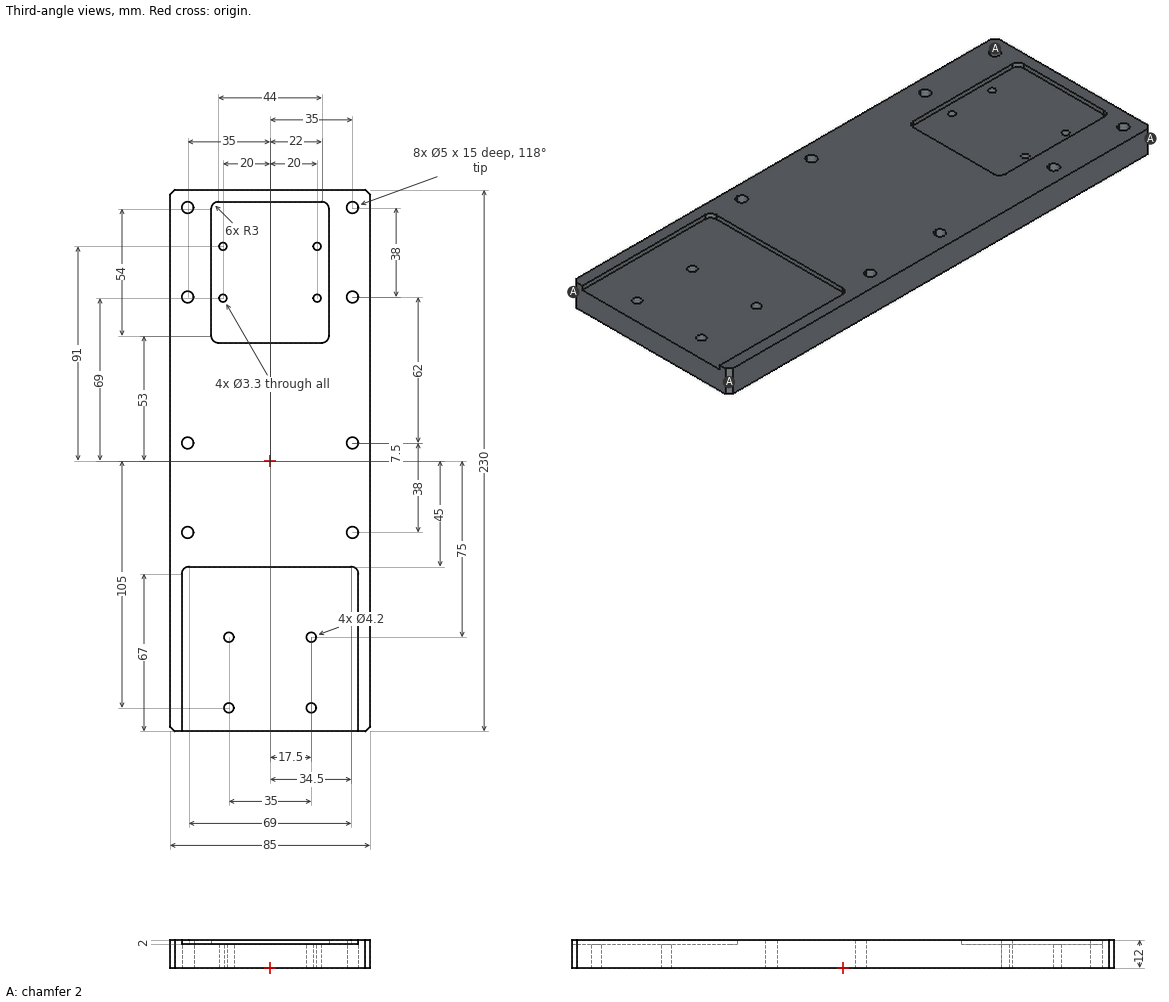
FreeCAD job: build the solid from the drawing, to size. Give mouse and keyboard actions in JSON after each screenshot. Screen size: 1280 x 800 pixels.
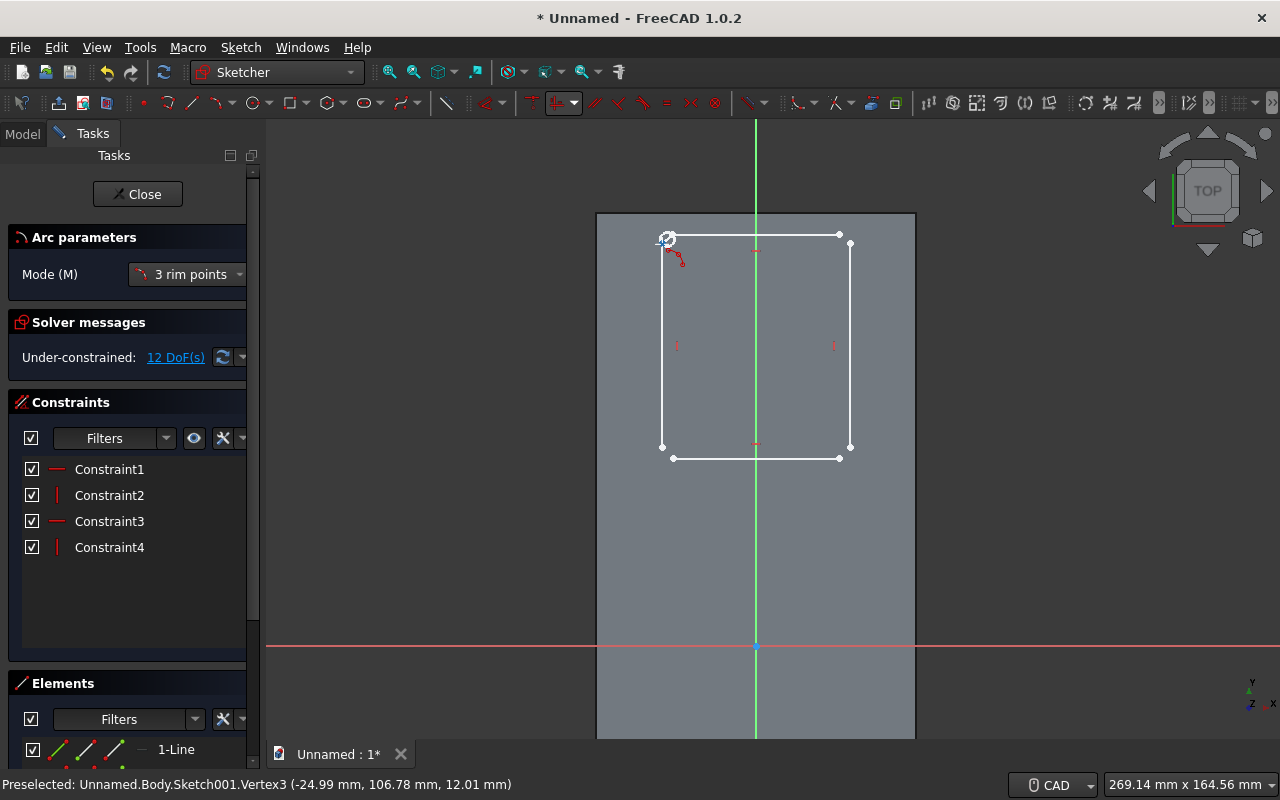
{"action": "scroll", "coordinate": [665, 235], "scroll_direction": "up", "scroll_amount": 8}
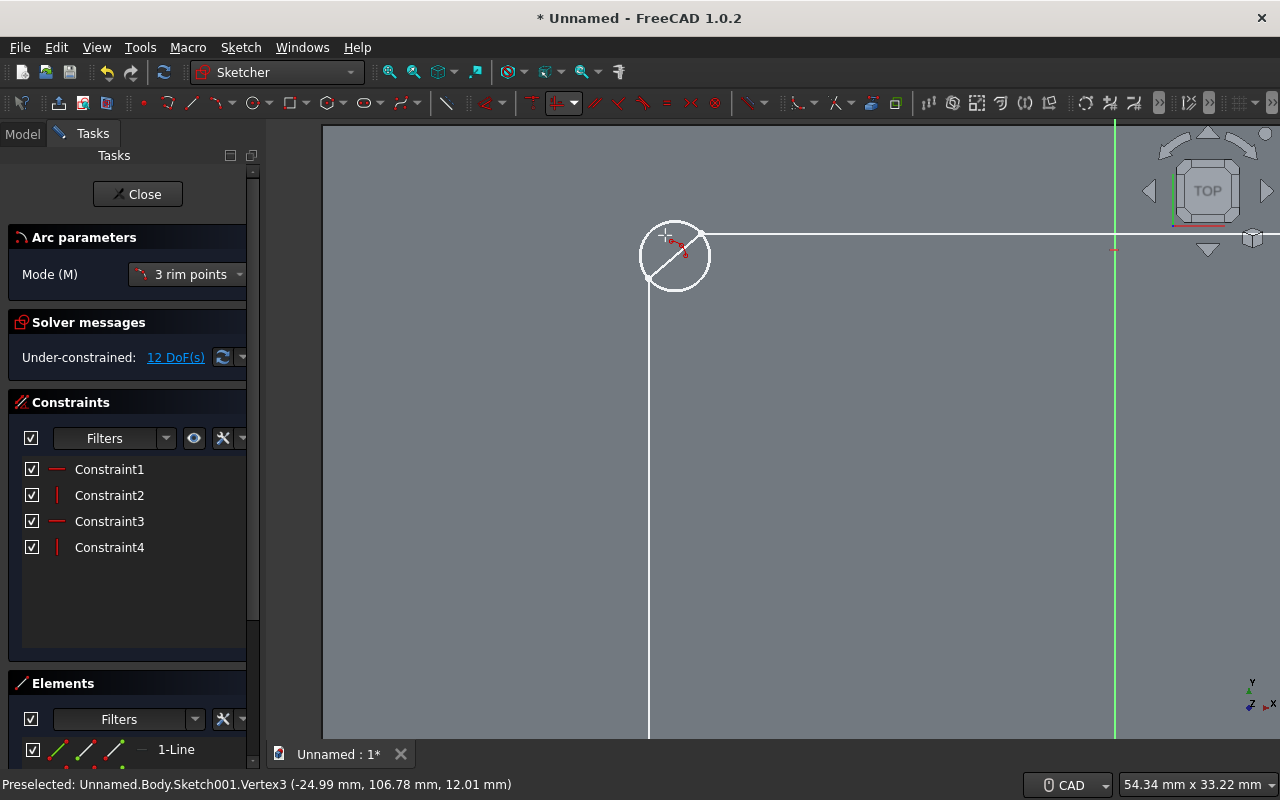
{"action": "left_click", "coordinate": [665, 235]}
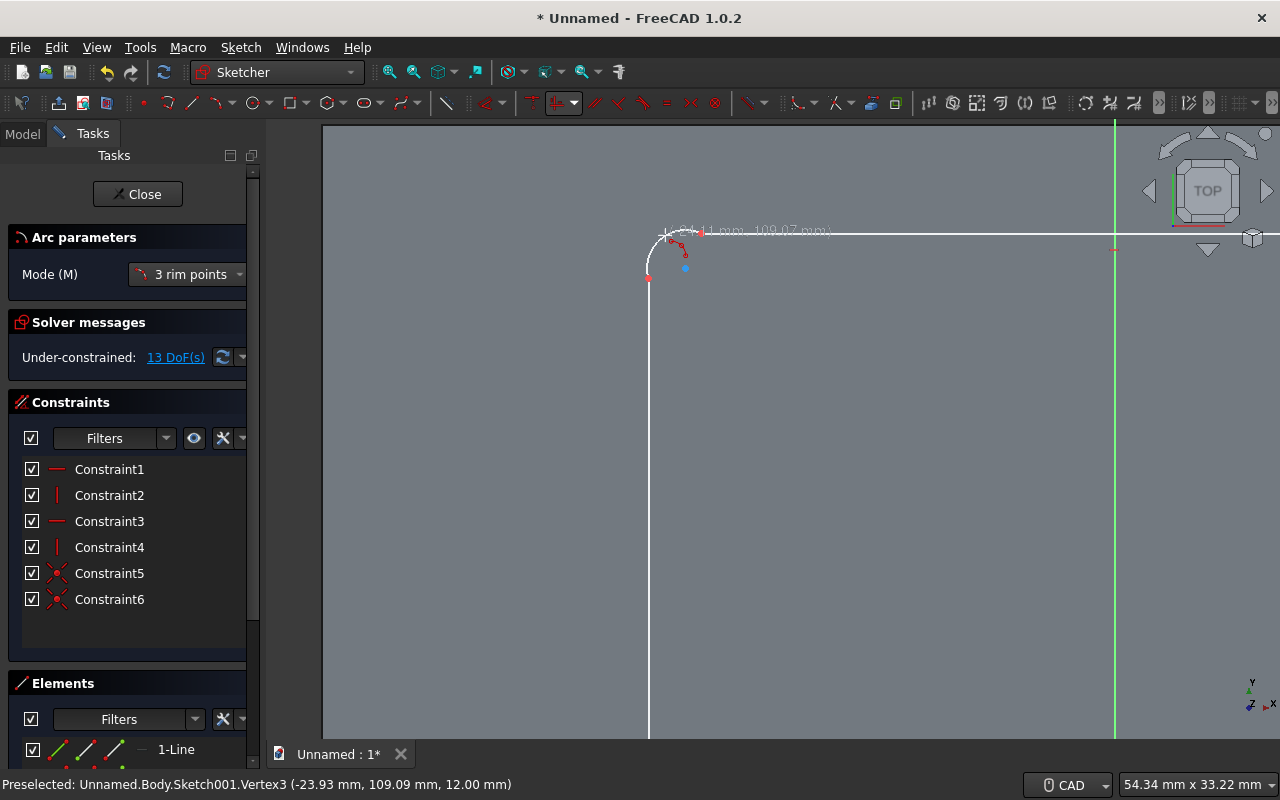
{"action": "scroll", "coordinate": [664, 241], "scroll_direction": "down", "scroll_amount": 12}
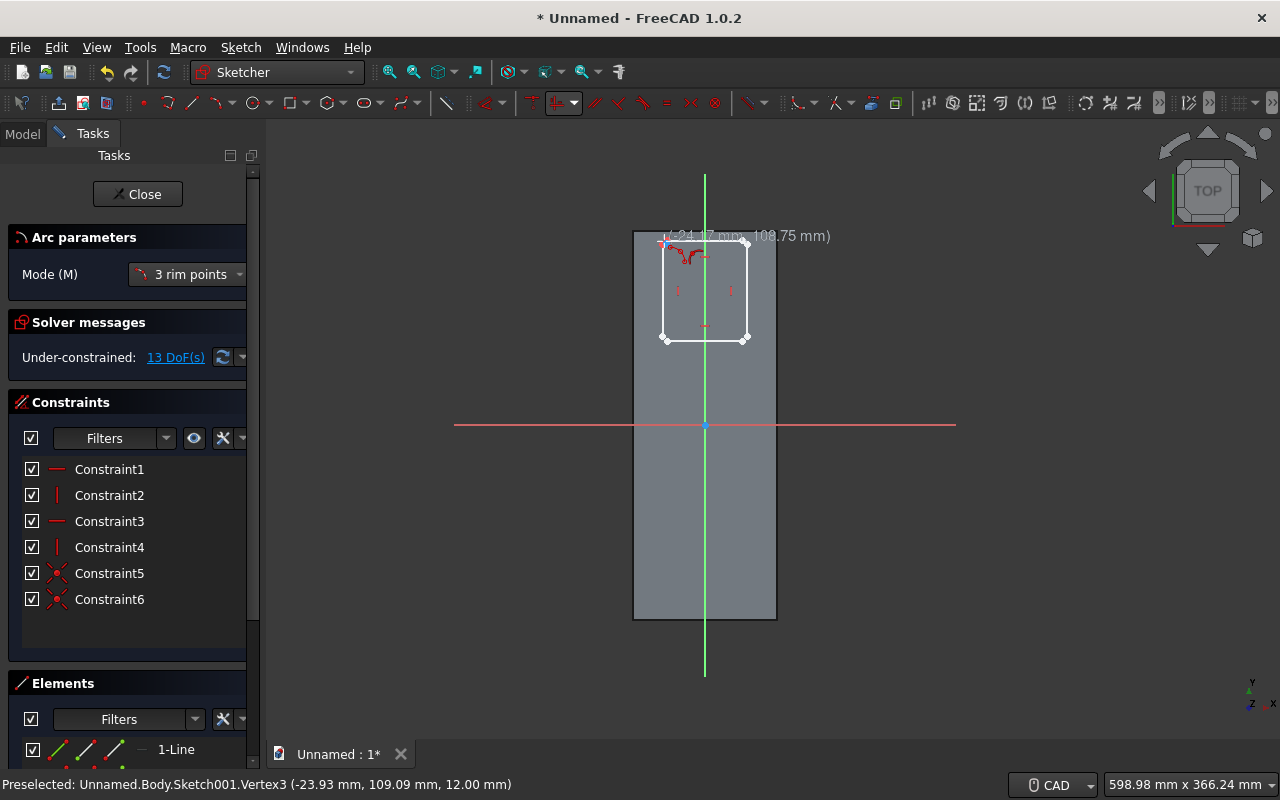
{"action": "scroll", "coordinate": [663, 336], "scroll_direction": "up", "scroll_amount": 4}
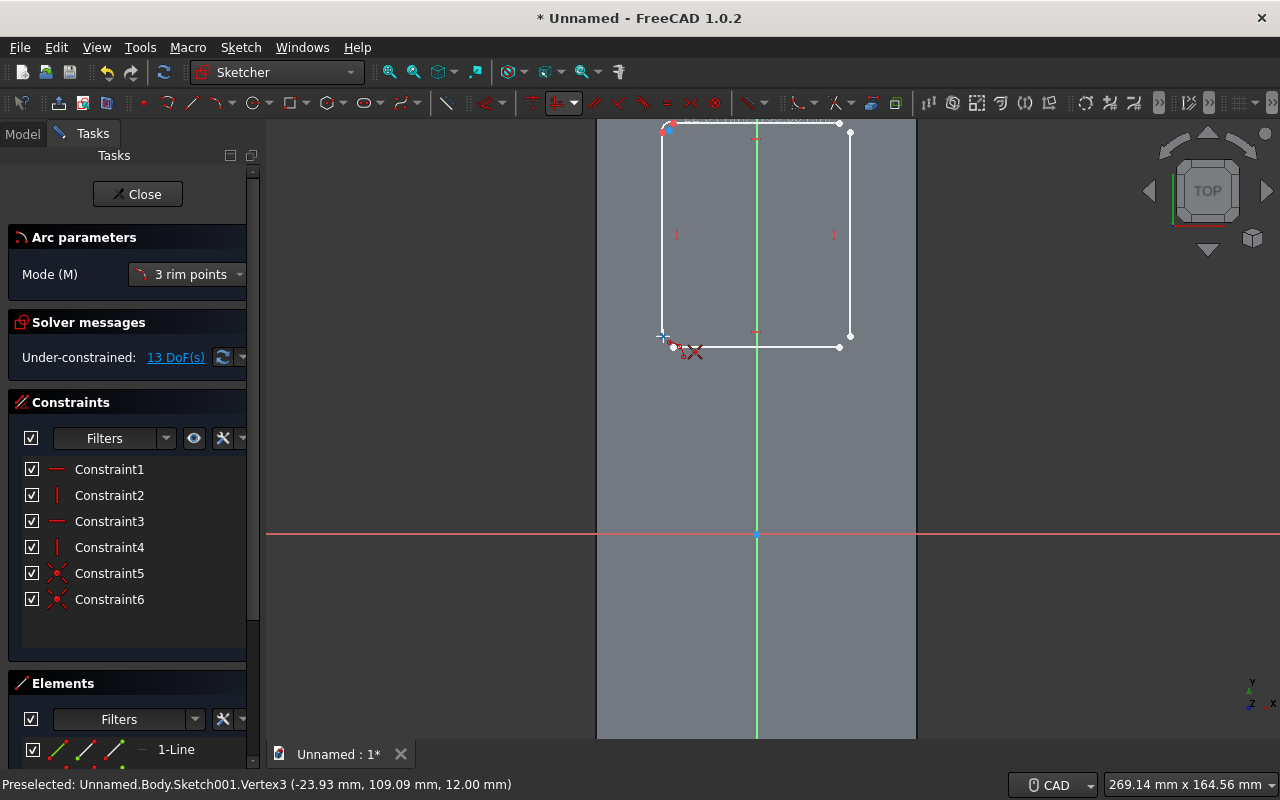
{"action": "left_click", "coordinate": [662, 336]}
{"action": "left_click", "coordinate": [673, 347]}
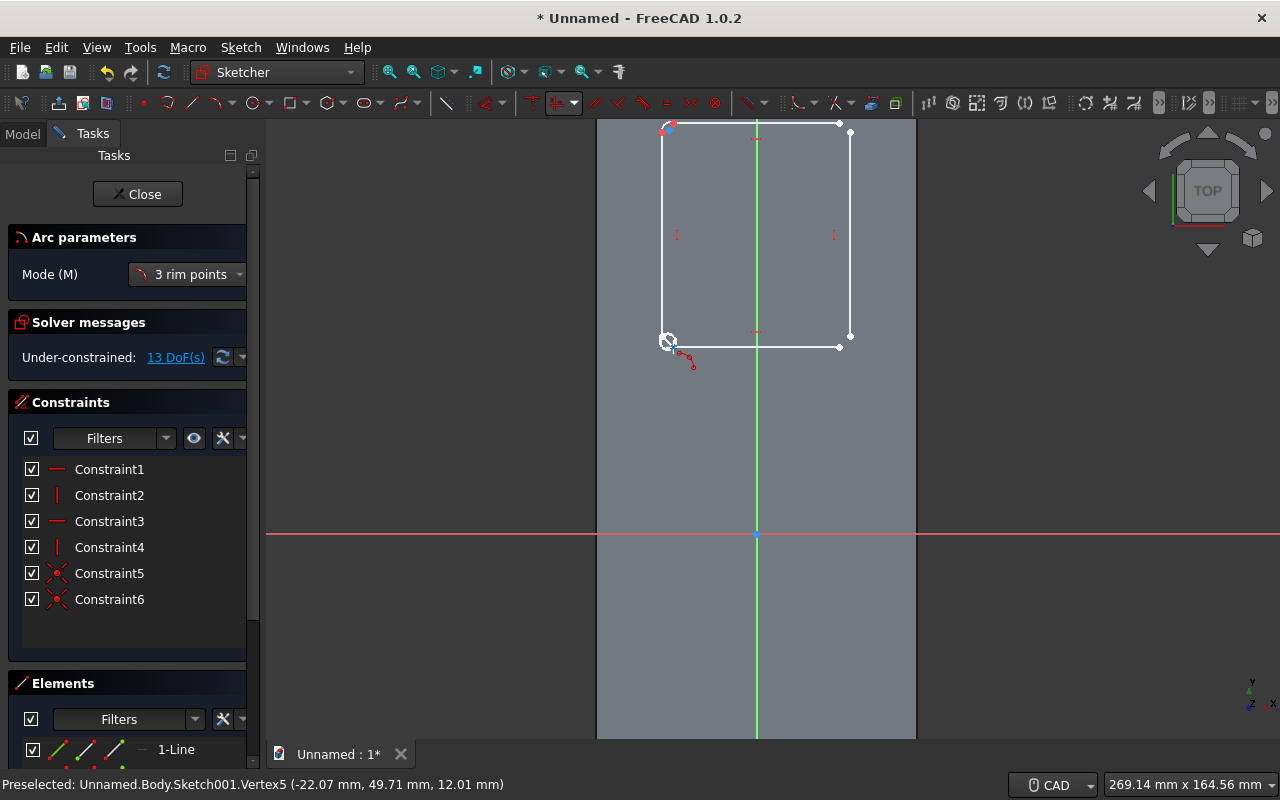
{"action": "scroll", "coordinate": [666, 343], "scroll_direction": "up", "scroll_amount": 8}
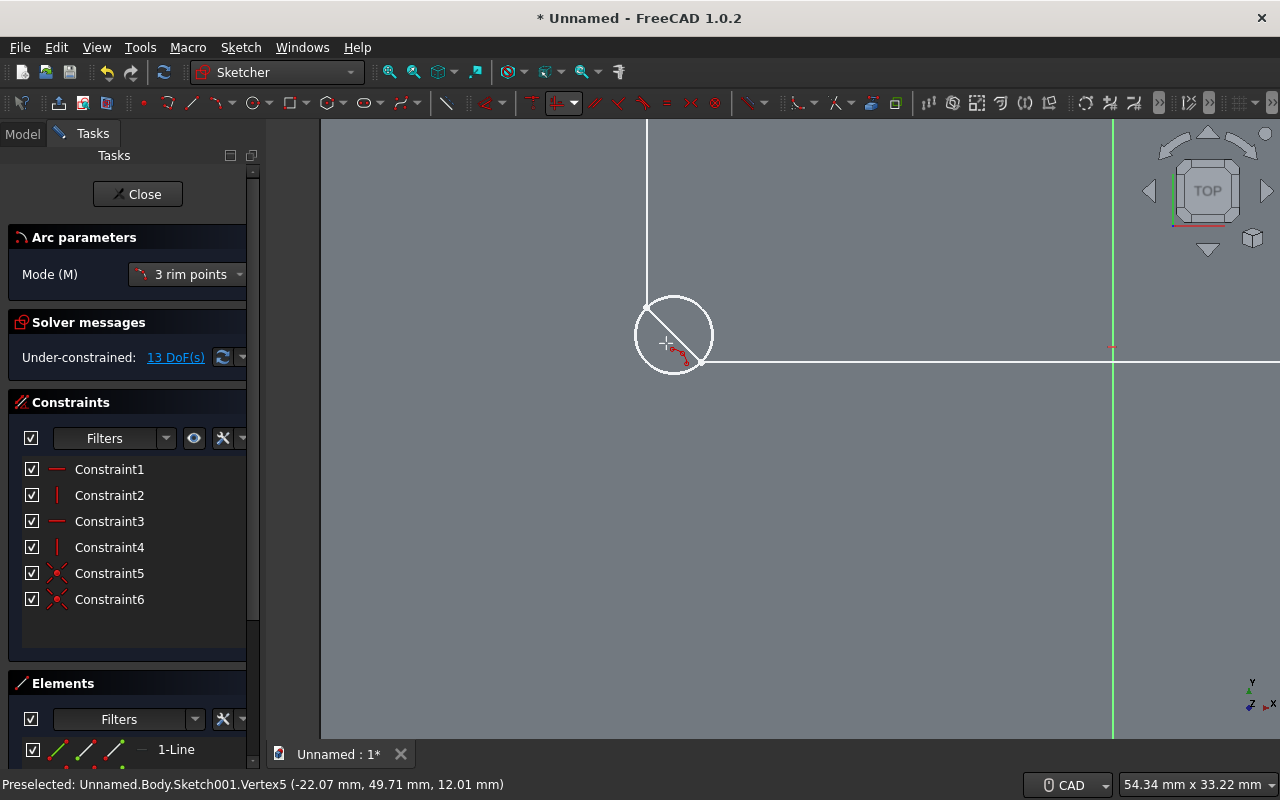
{"action": "left_click", "coordinate": [663, 340]}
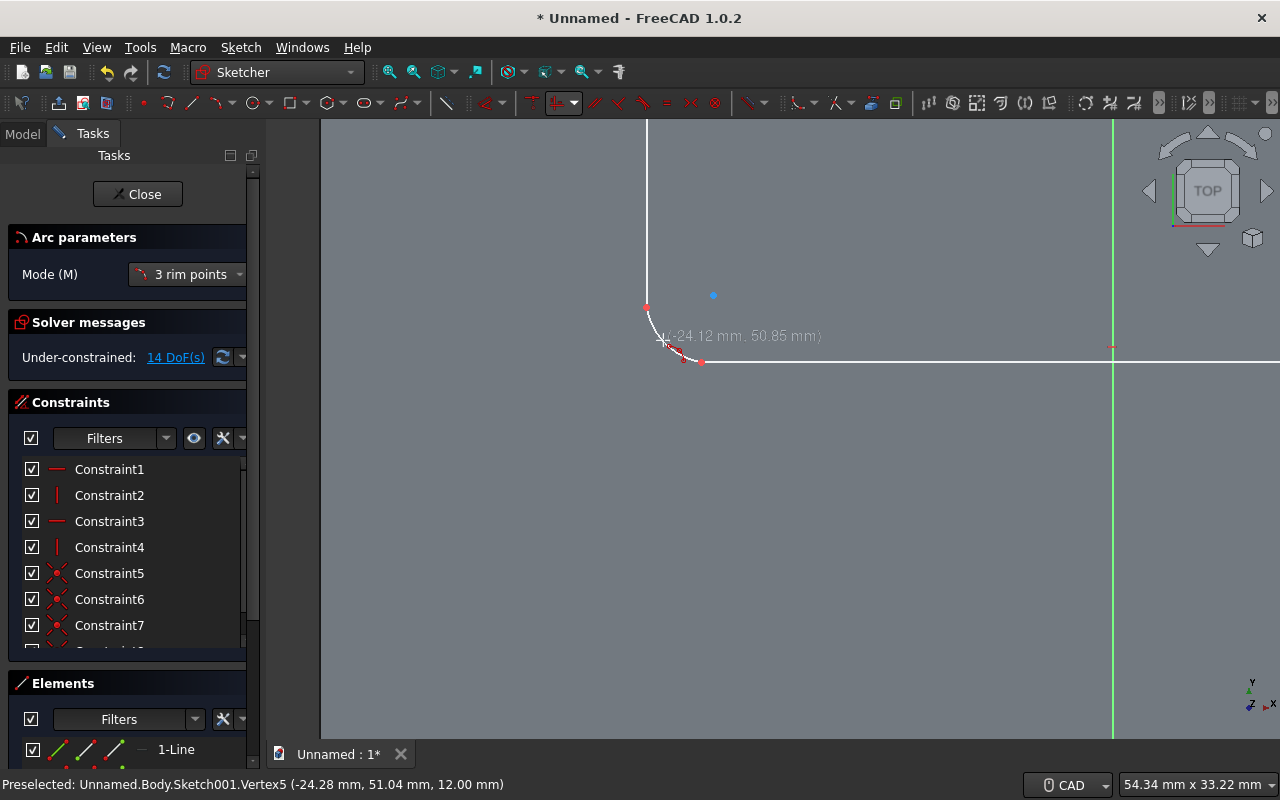
{"action": "scroll", "coordinate": [664, 338], "scroll_direction": "down", "scroll_amount": 12}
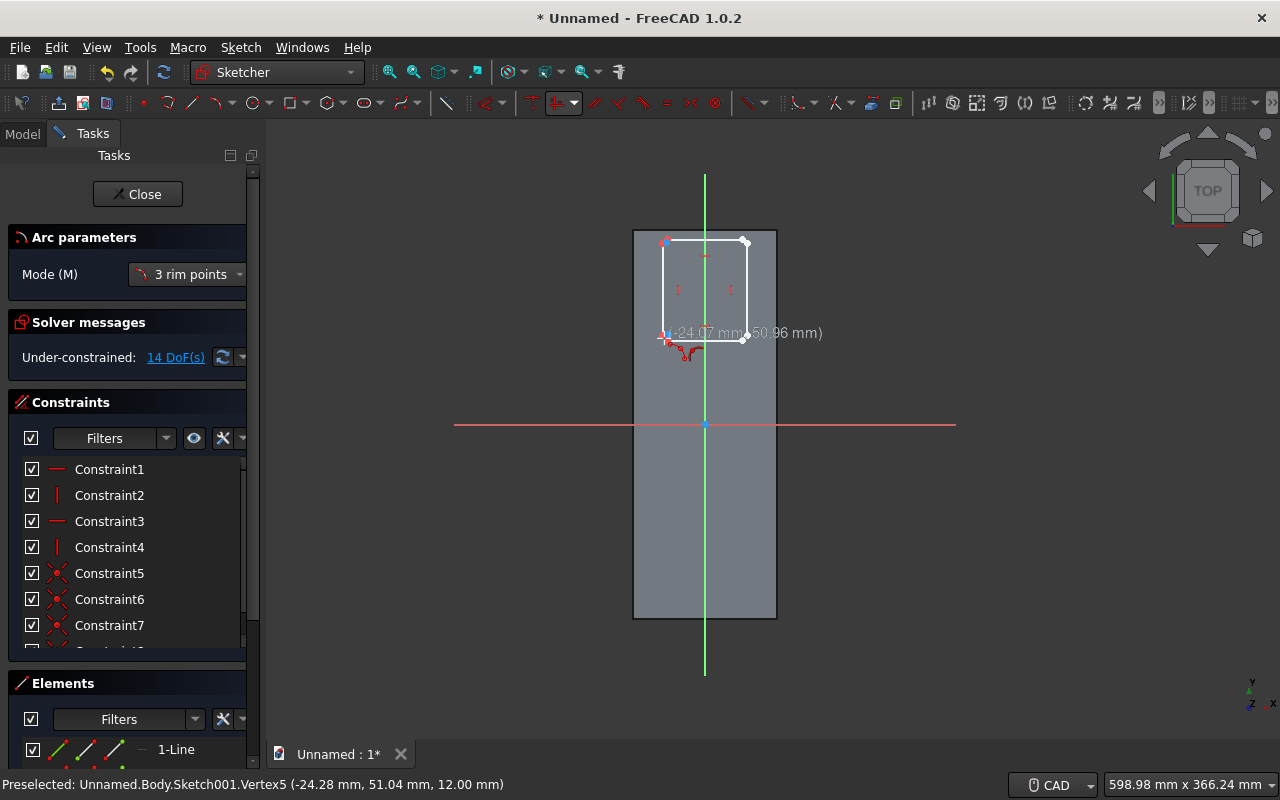
{"action": "scroll", "coordinate": [742, 340], "scroll_direction": "up", "scroll_amount": 4}